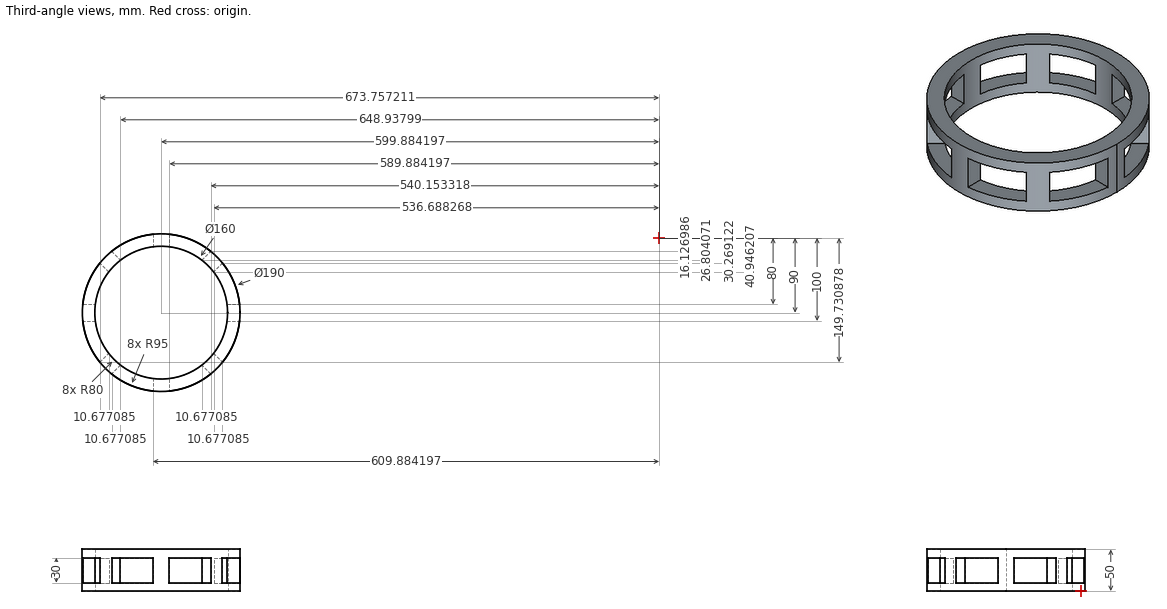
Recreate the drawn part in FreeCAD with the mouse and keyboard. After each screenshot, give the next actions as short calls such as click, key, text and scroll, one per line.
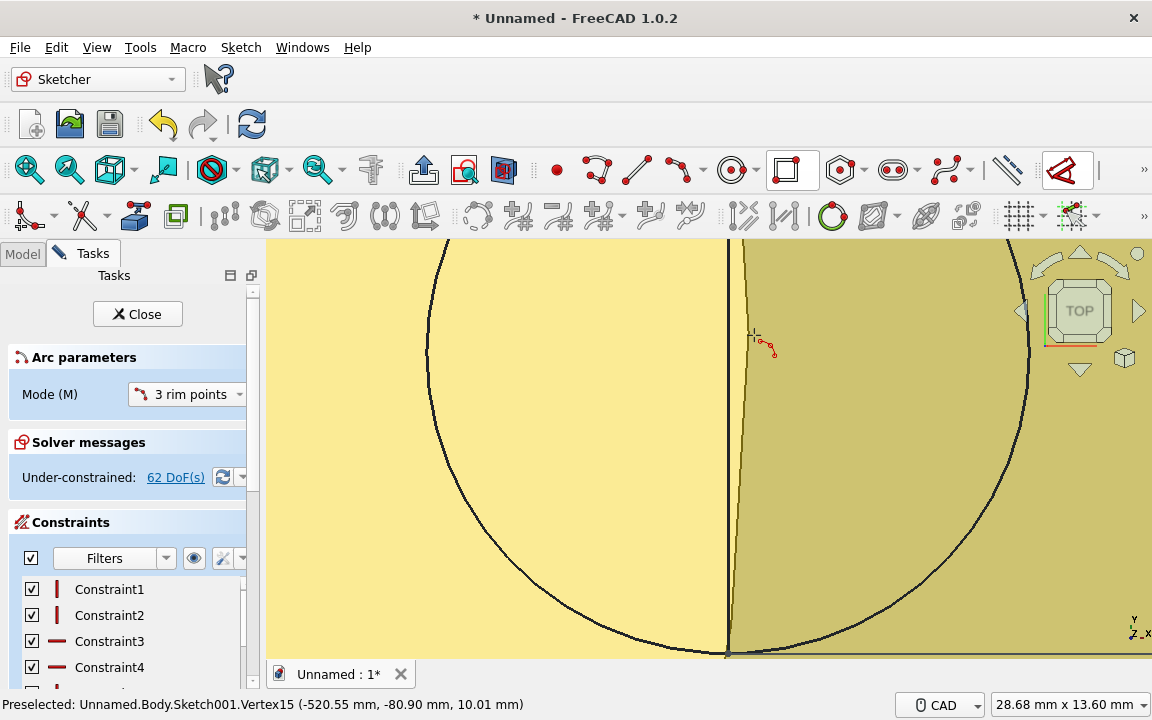
click(749, 332)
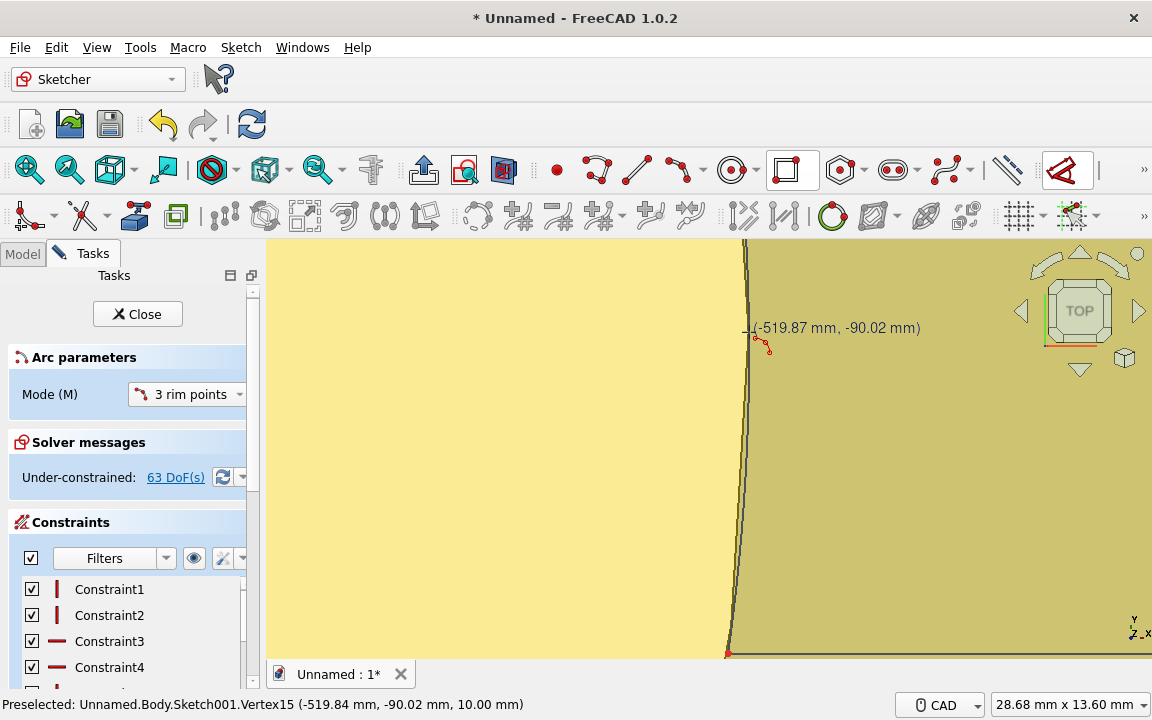
scroll(764, 455, down, 15)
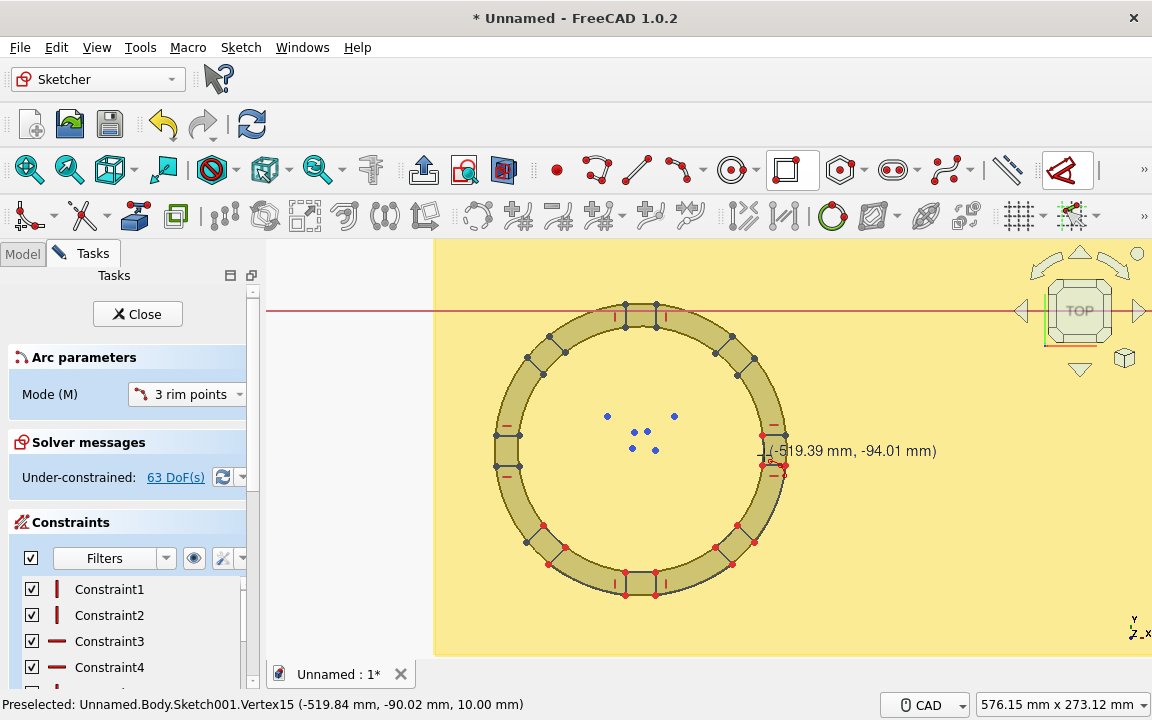
scroll(786, 434, up, 2)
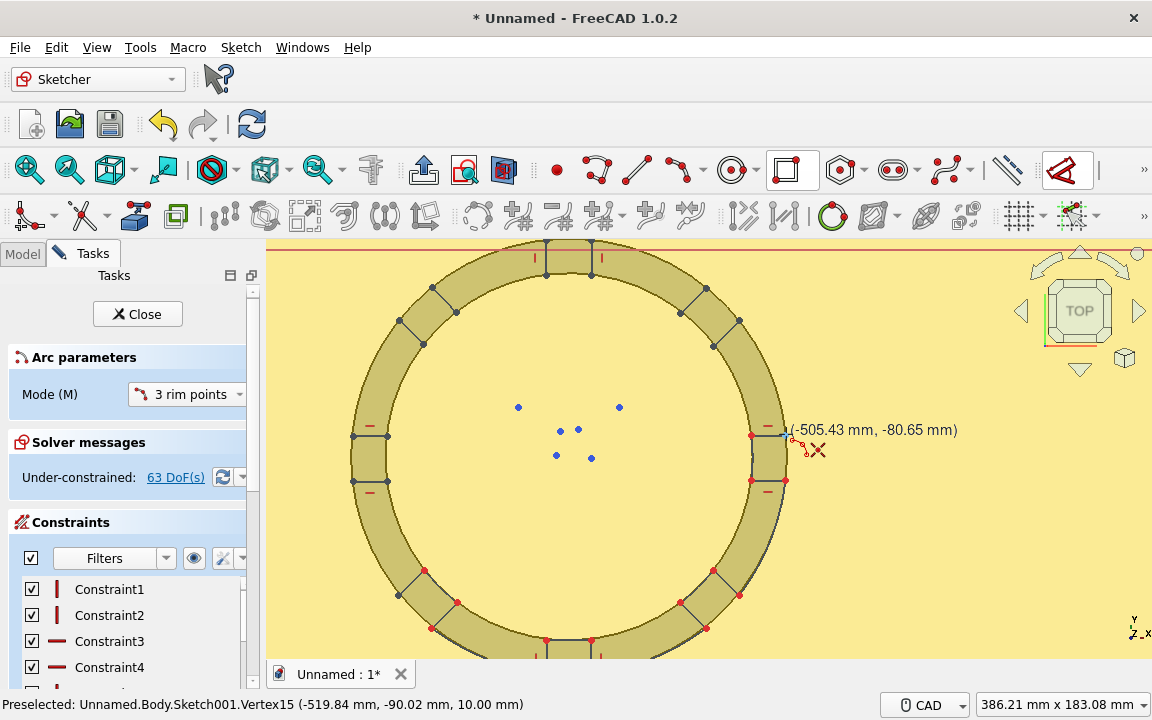
click(785, 436)
click(739, 321)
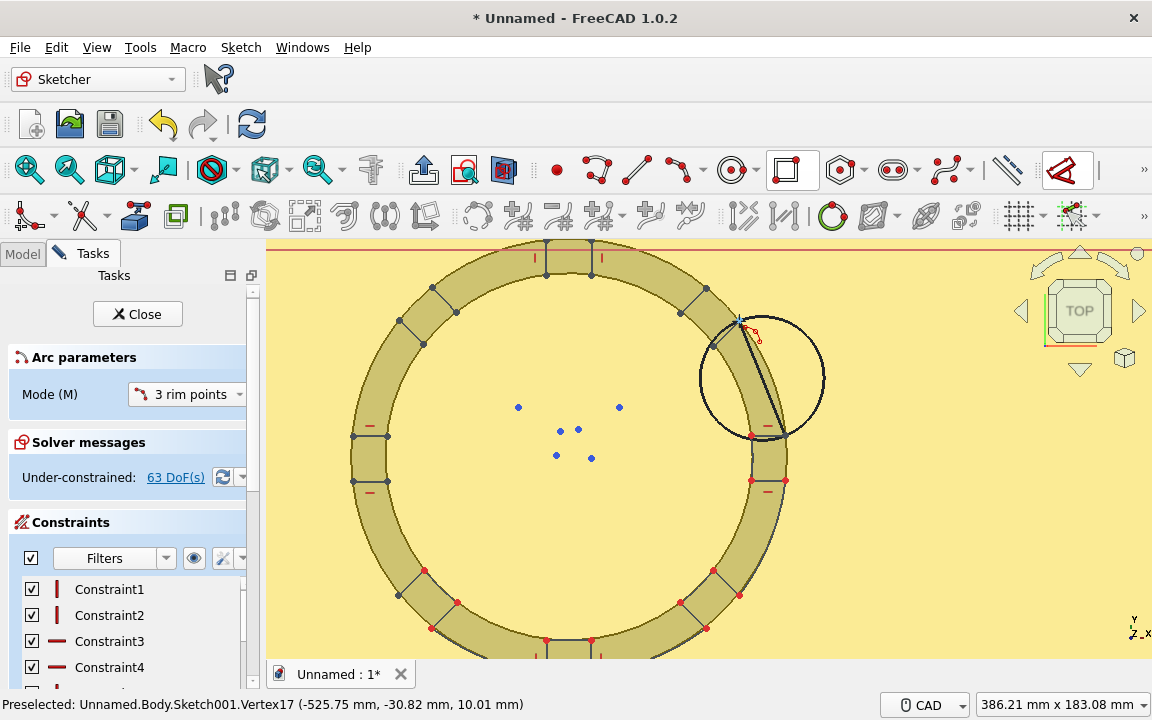
scroll(770, 373, up, 3)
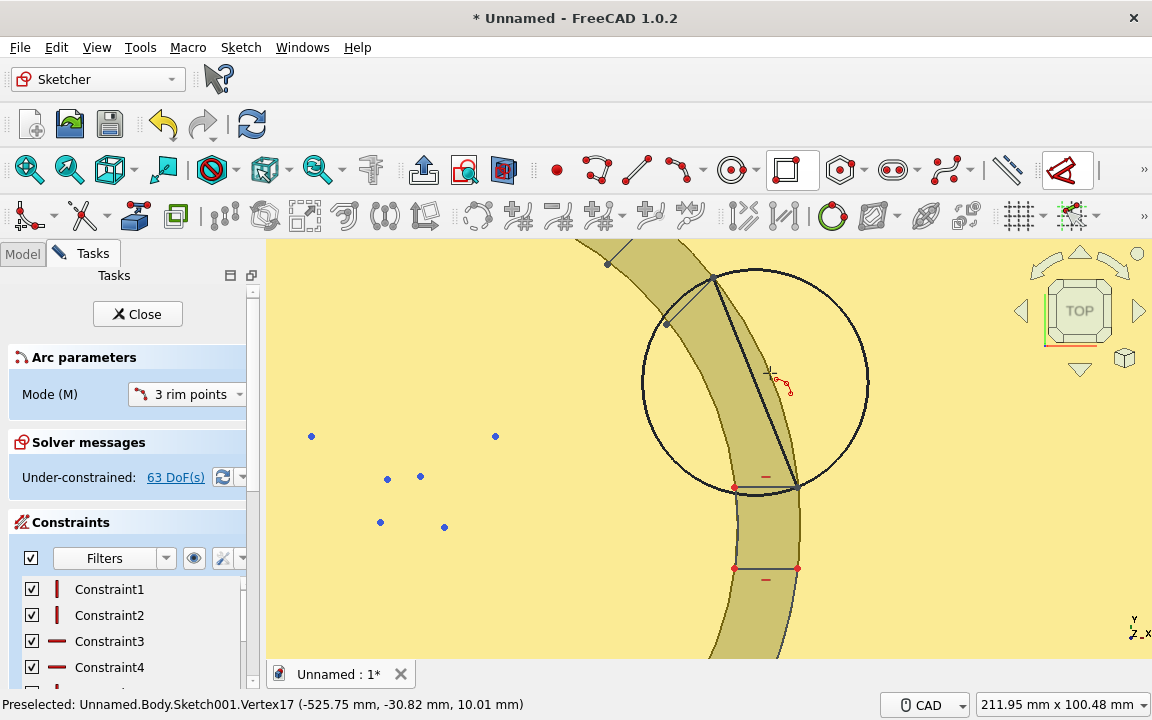
click(770, 373)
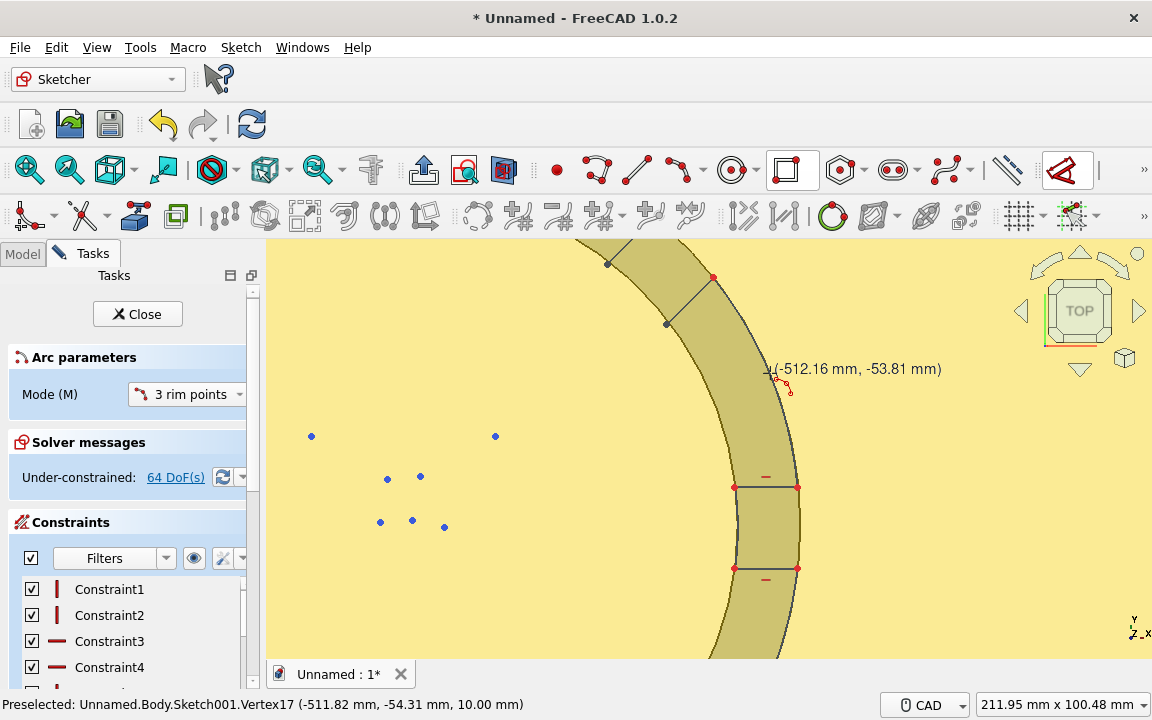
click(667, 324)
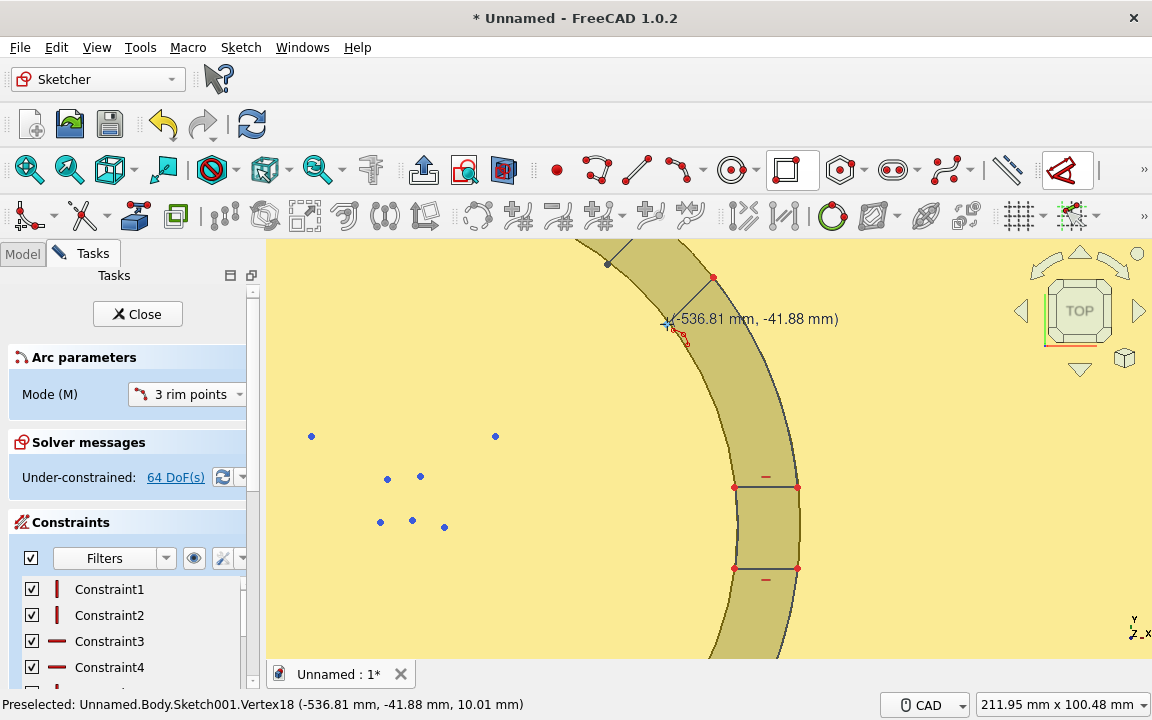
scroll(743, 416, down, 6)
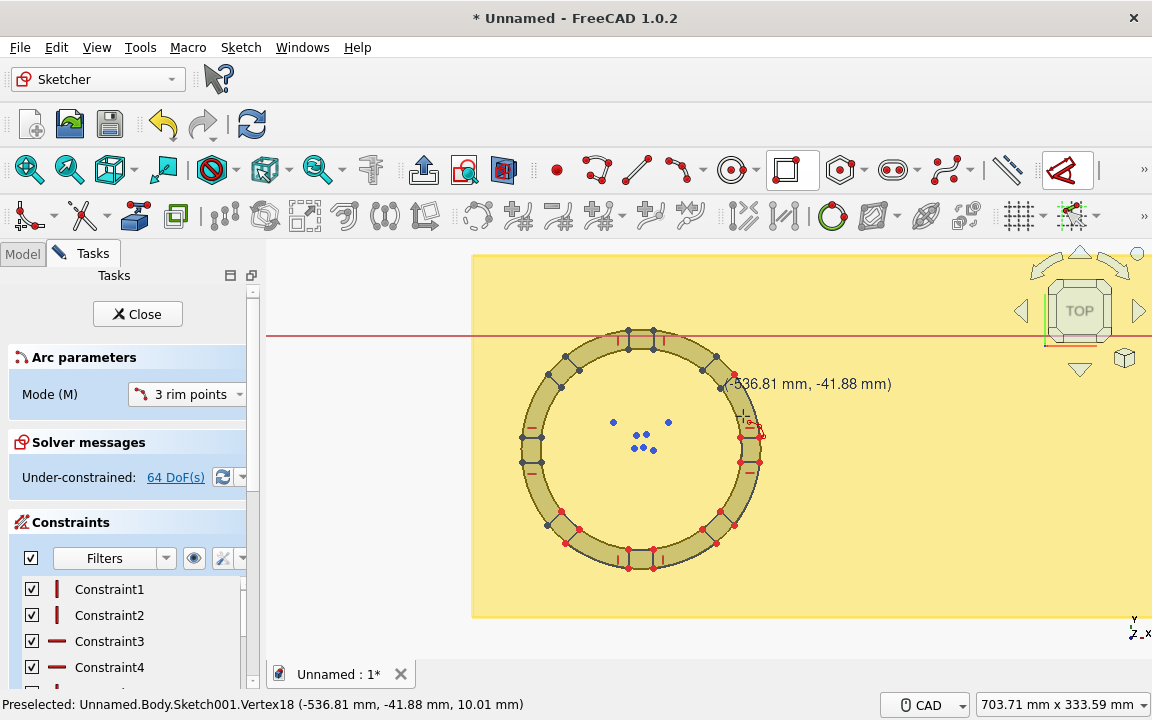
scroll(703, 370, up, 3)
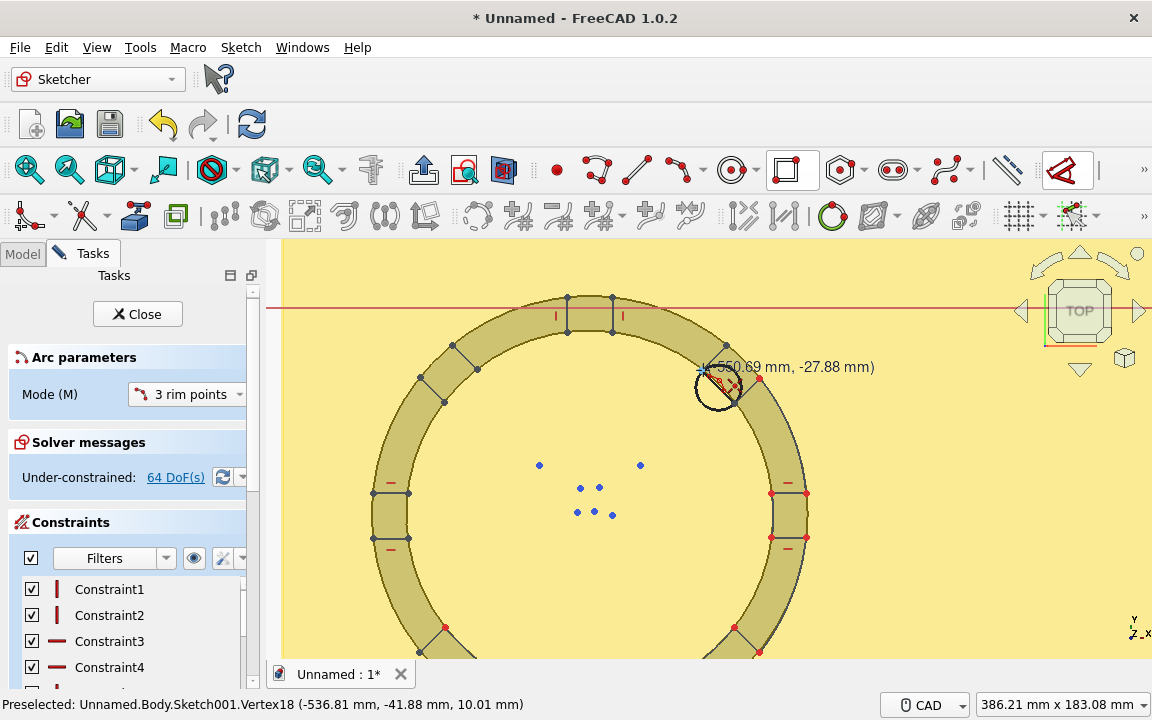
click(702, 371)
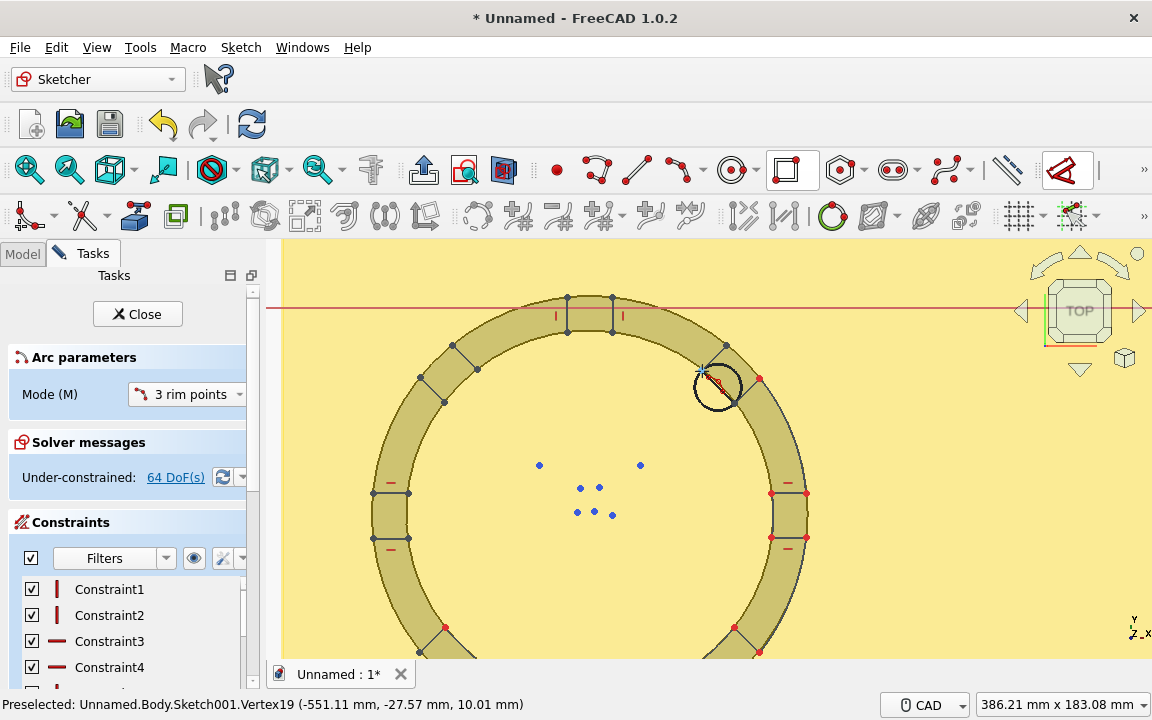
scroll(720, 384, up, 13)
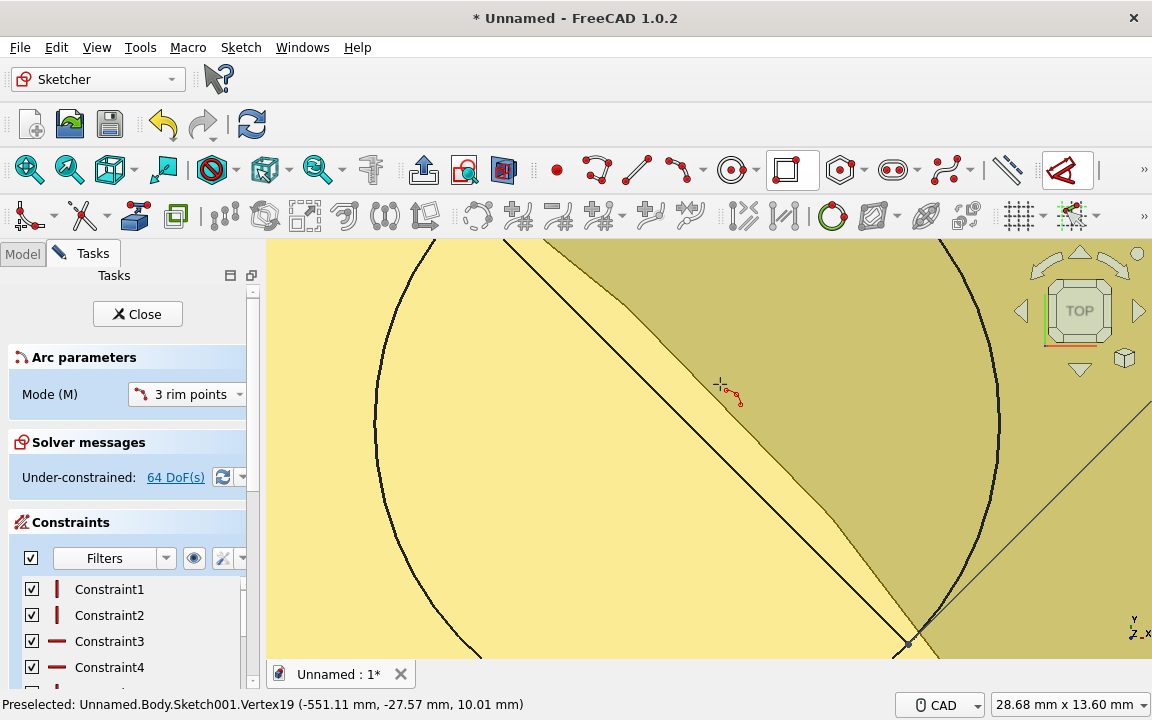
click(707, 384)